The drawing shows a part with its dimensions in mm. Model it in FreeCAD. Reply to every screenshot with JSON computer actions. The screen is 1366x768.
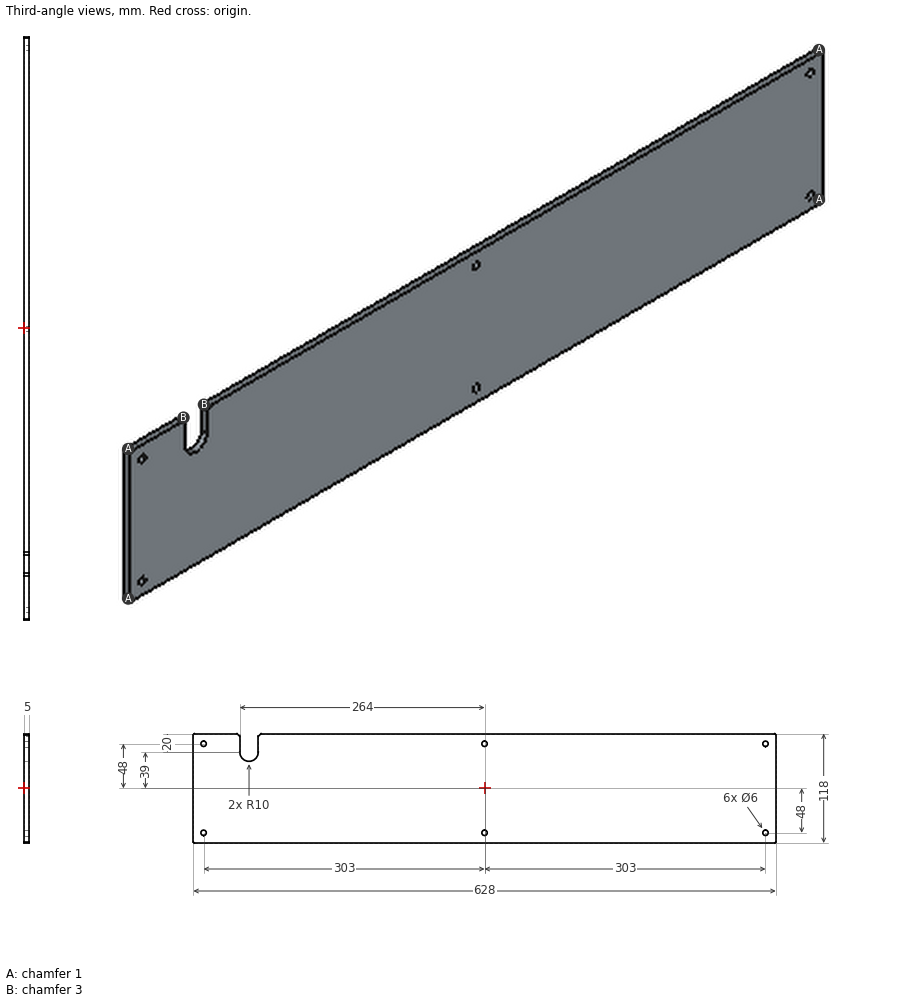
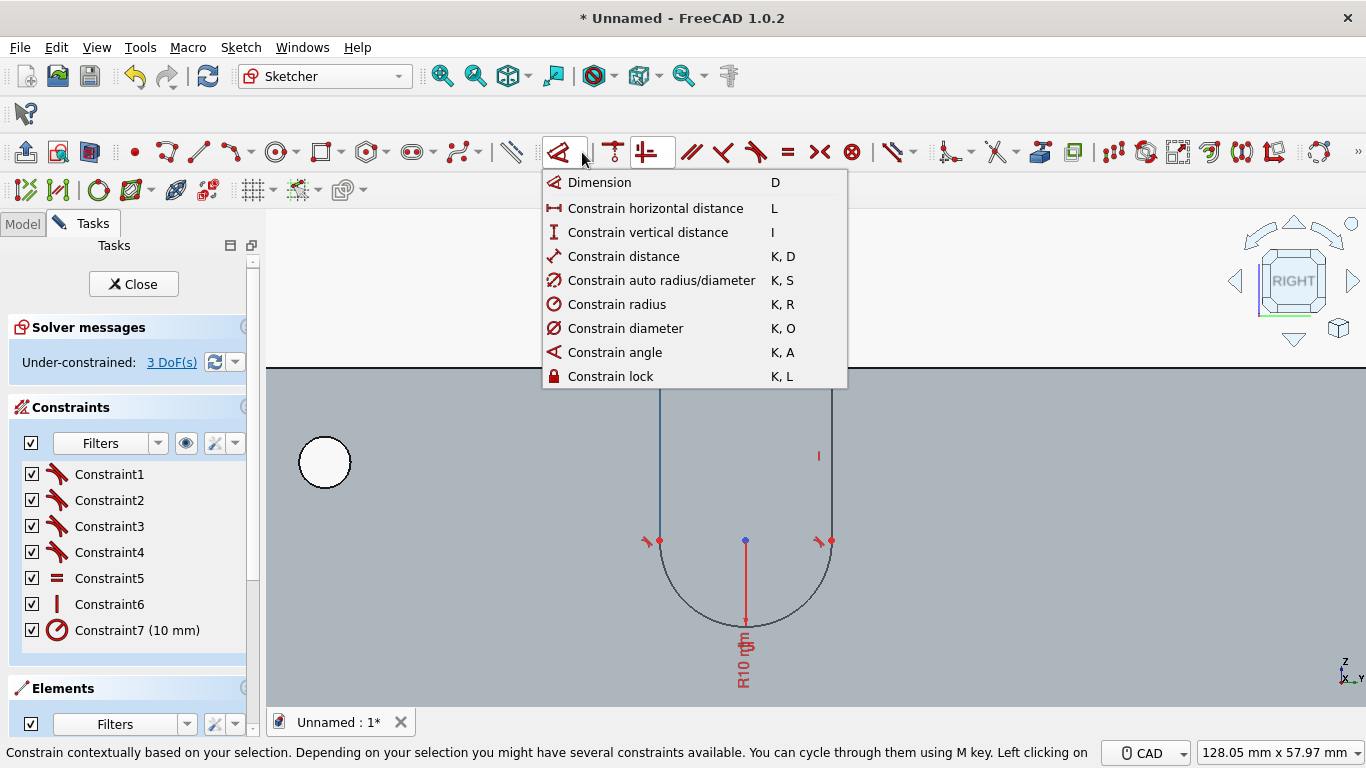
{"action": "left_click", "coordinate": [695, 232]}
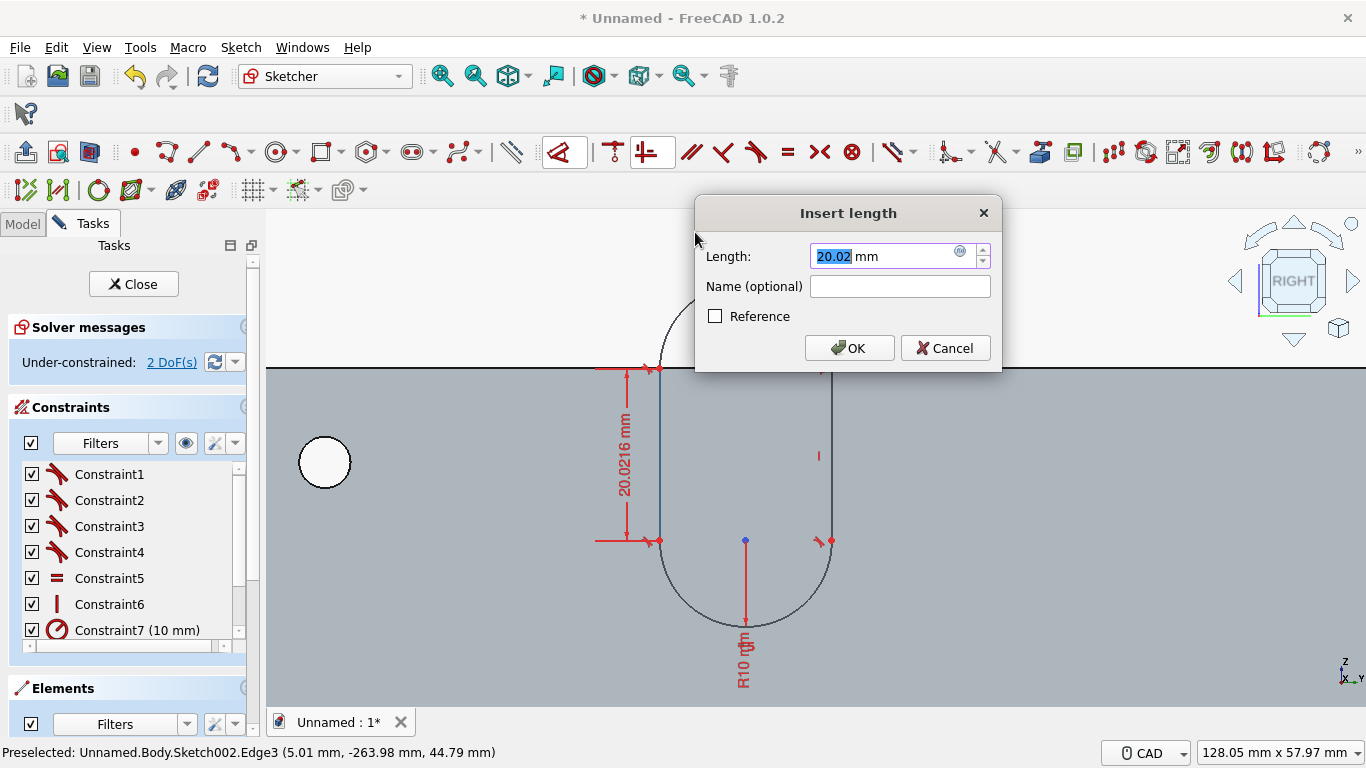
{"action": "type", "text": "20"}
{"action": "key", "text": "Return"}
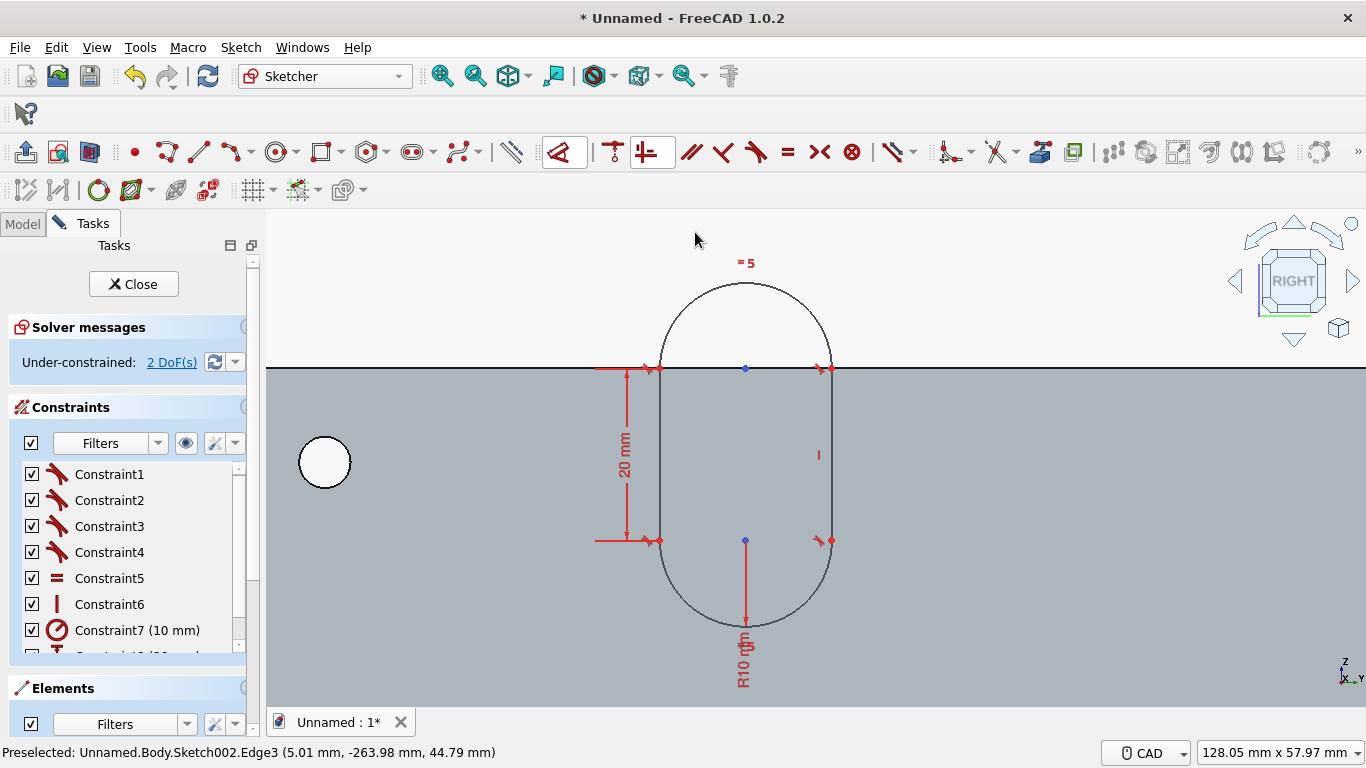
{"action": "left_click", "coordinate": [660, 541]}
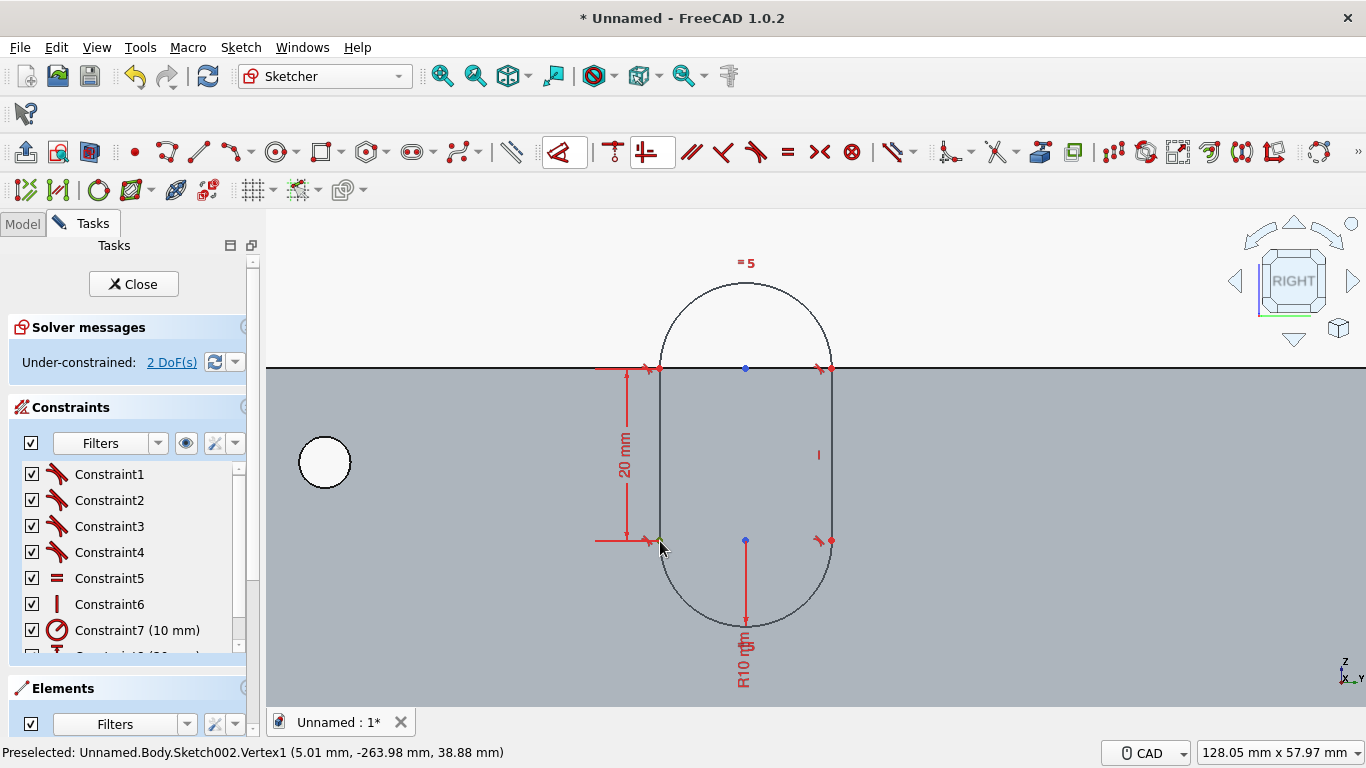
{"action": "left_click", "coordinate": [582, 152]}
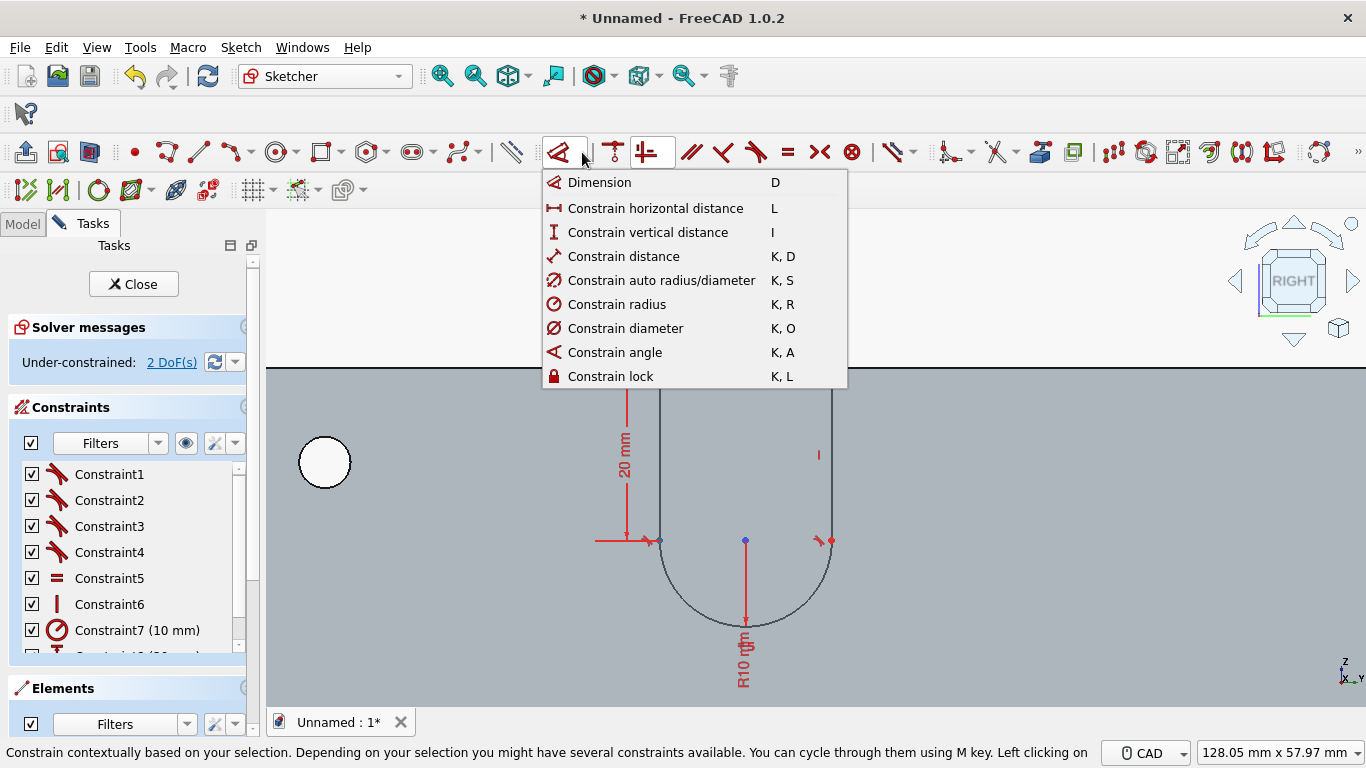
{"action": "left_click", "coordinate": [695, 232]}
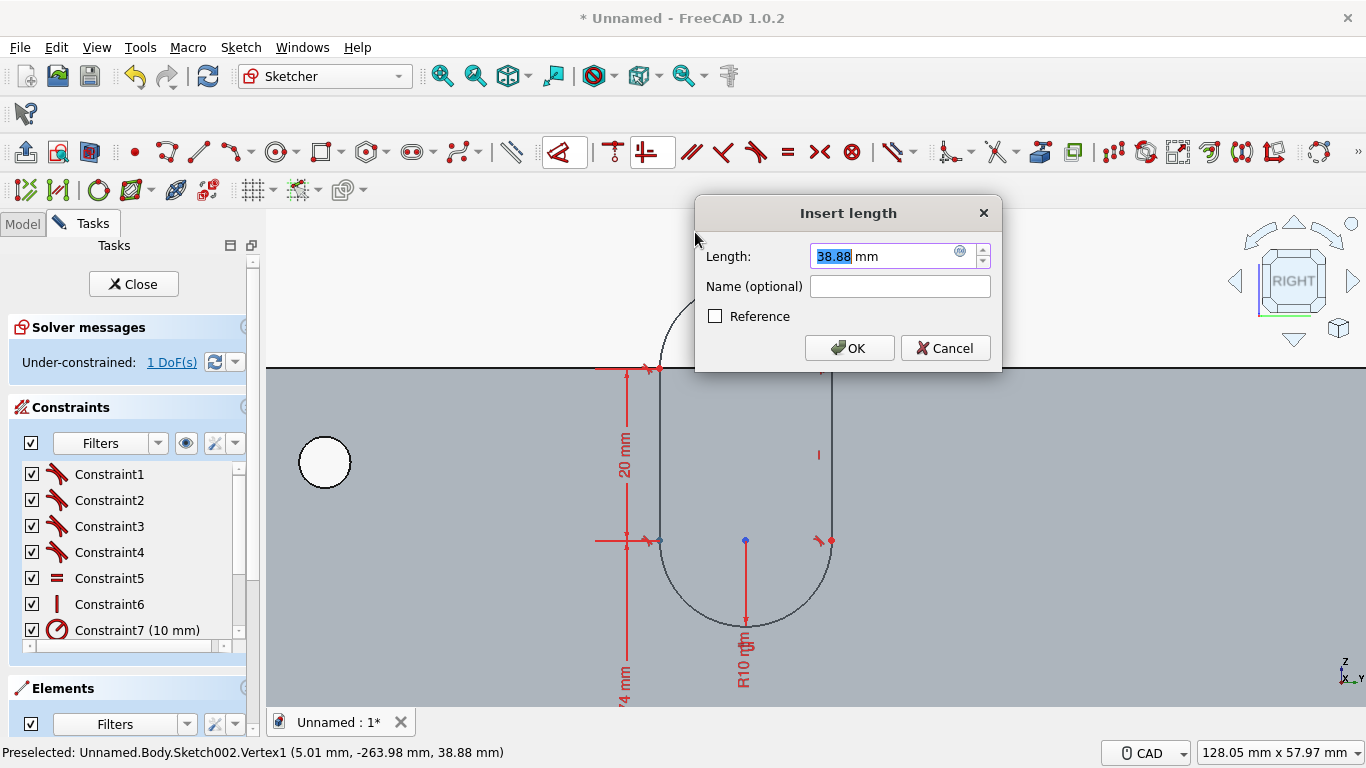
{"action": "type", "text": "39"}
{"action": "key", "text": "Return"}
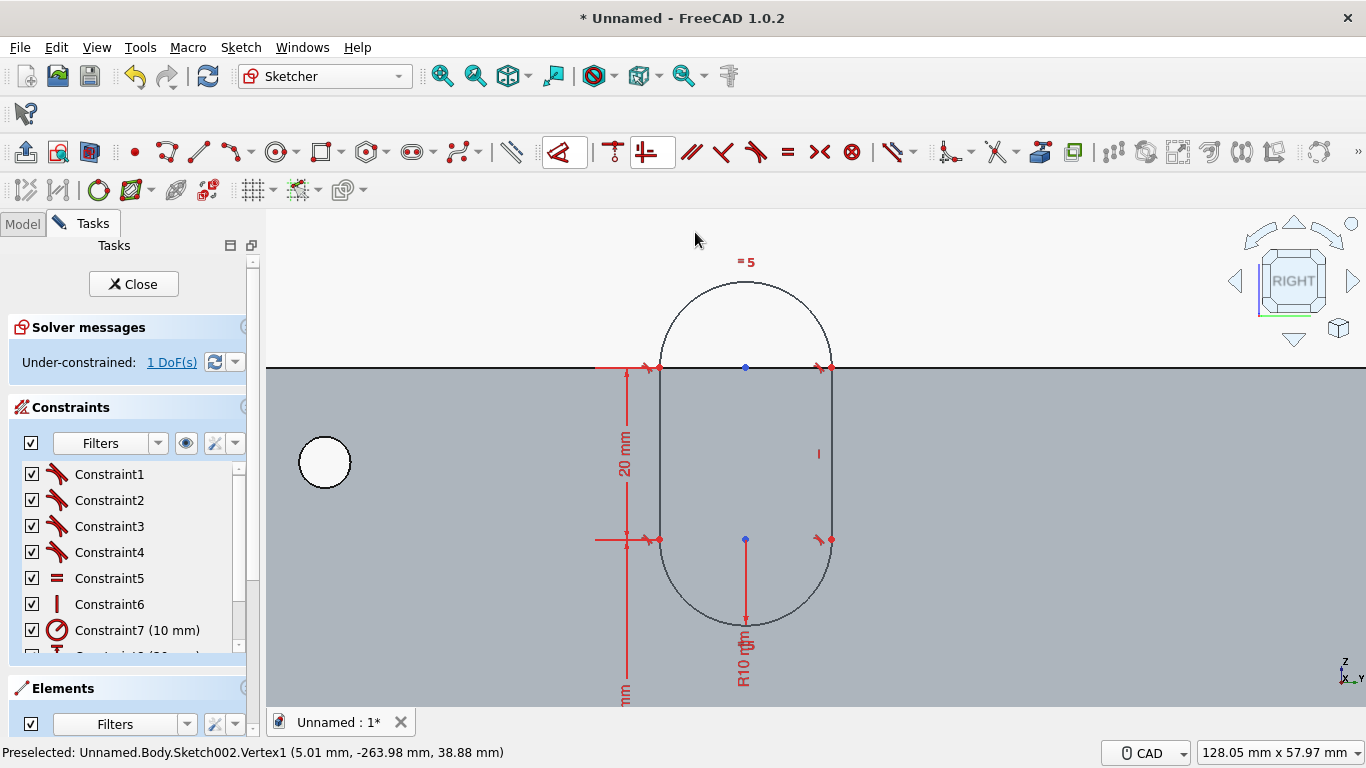
{"action": "left_click", "coordinate": [660, 540]}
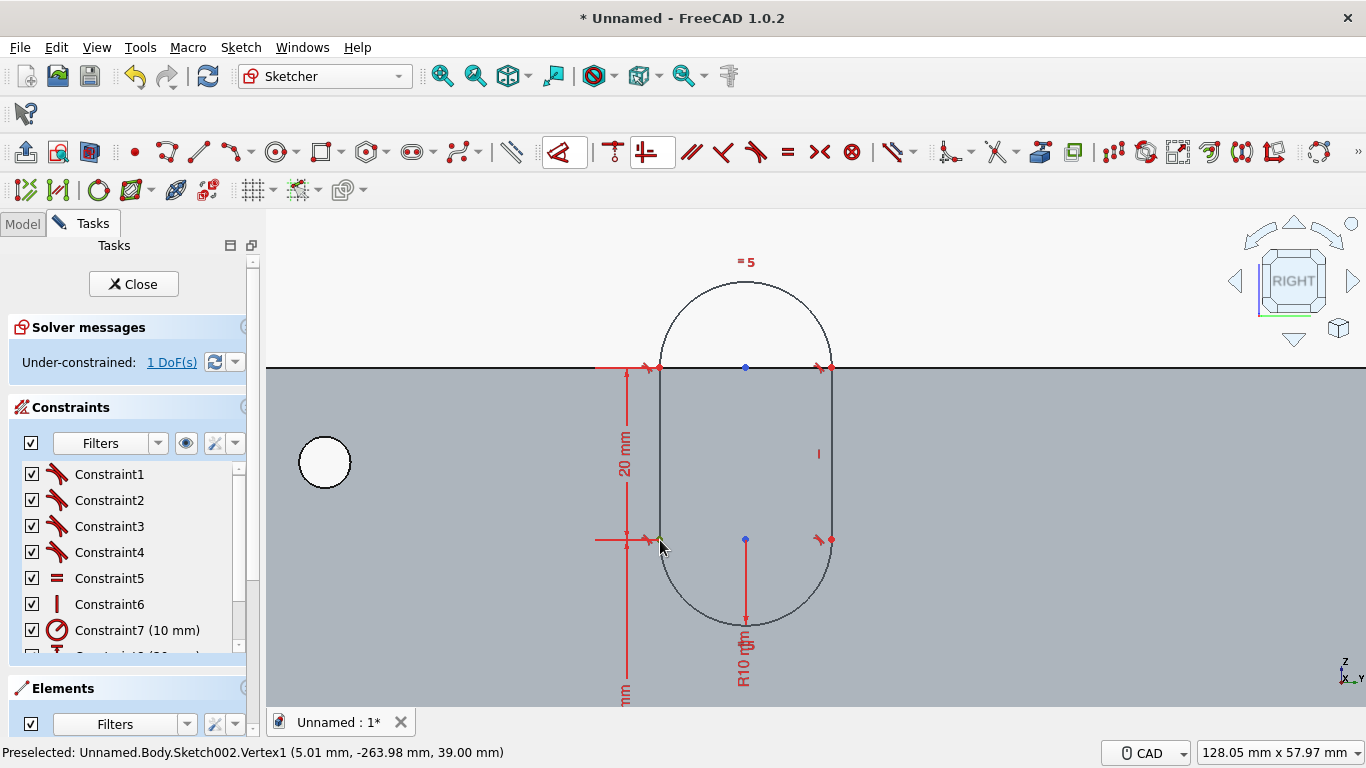
{"action": "left_click", "coordinate": [582, 152]}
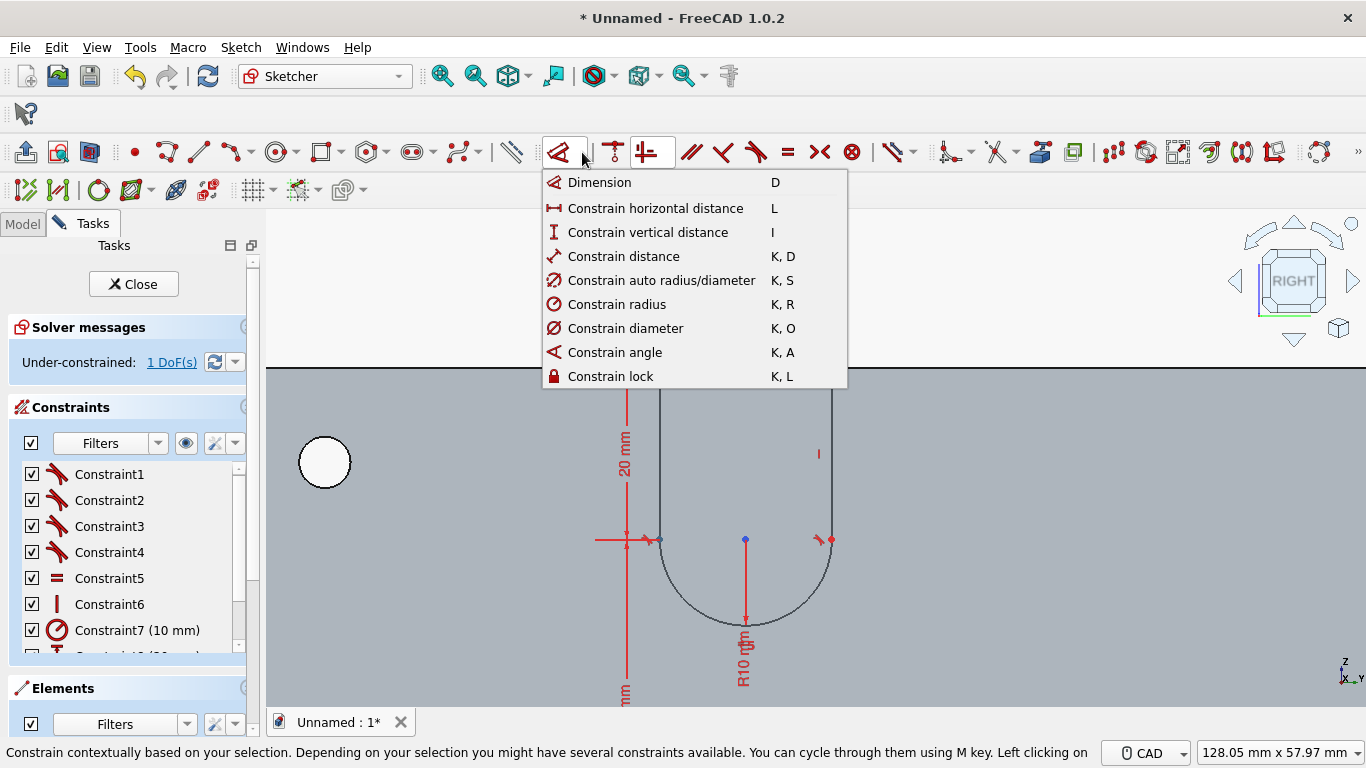
{"action": "left_click", "coordinate": [695, 208]}